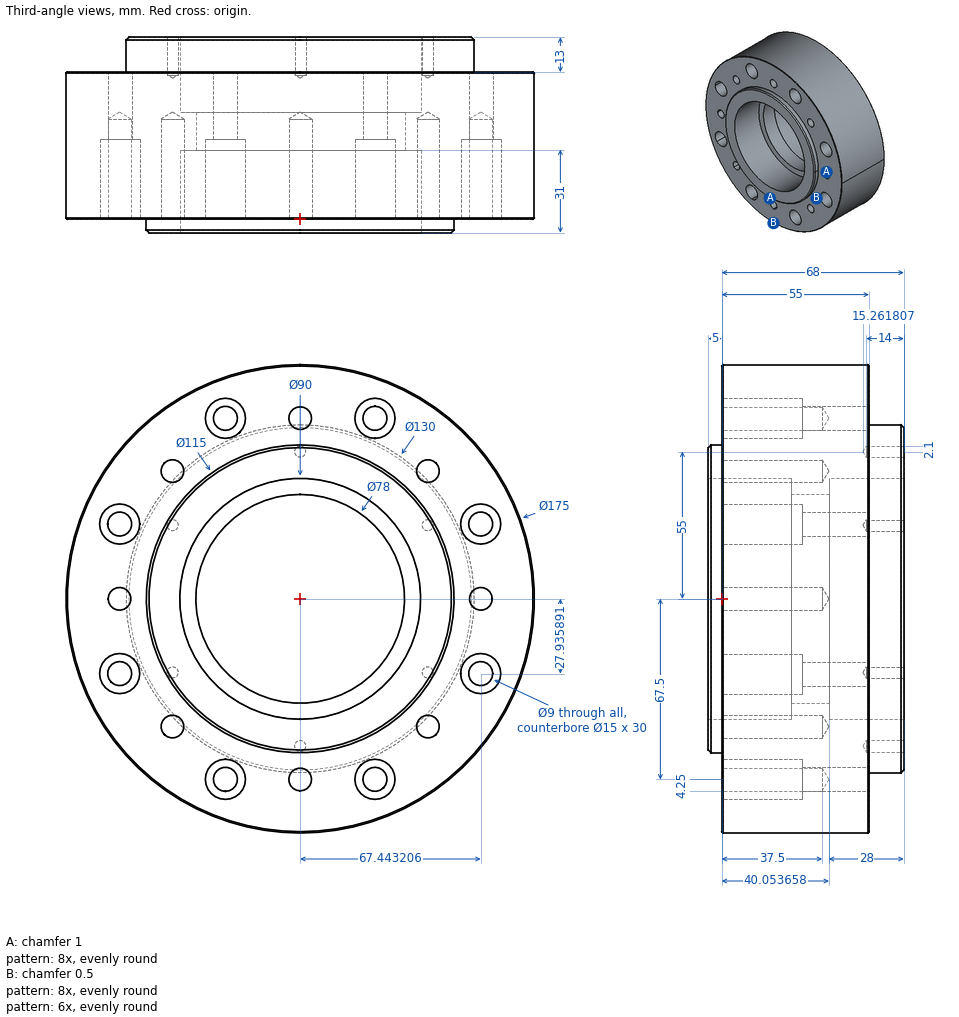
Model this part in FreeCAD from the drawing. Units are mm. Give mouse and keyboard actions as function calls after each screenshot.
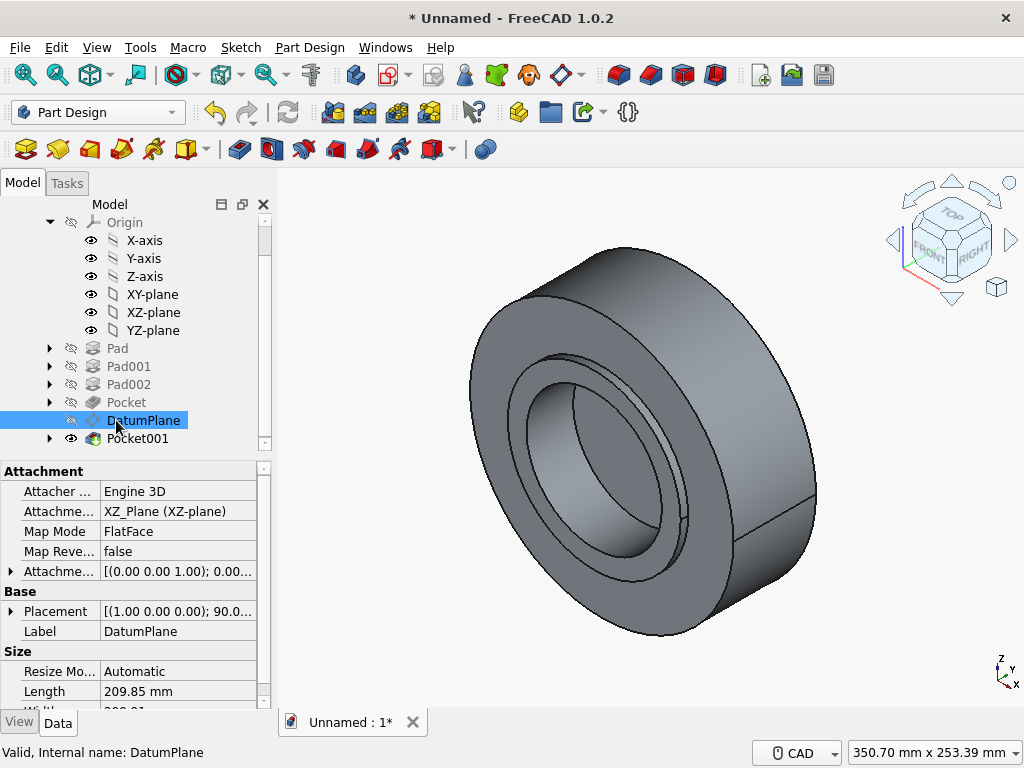
key(4)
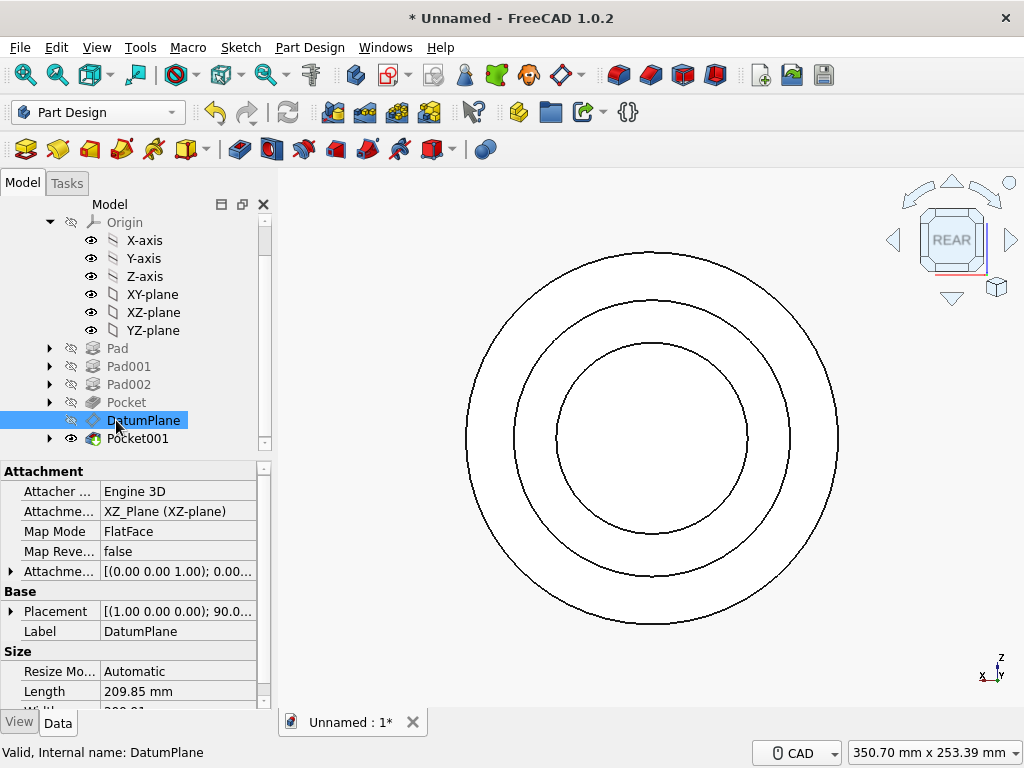
click(652, 437)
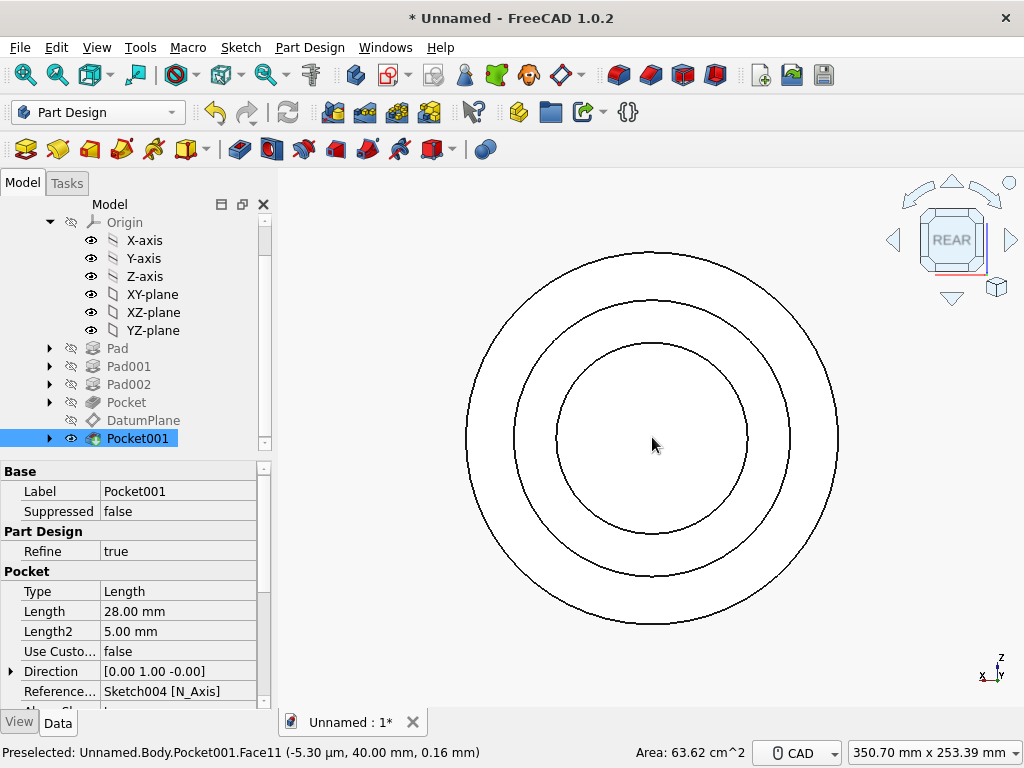
click(388, 76)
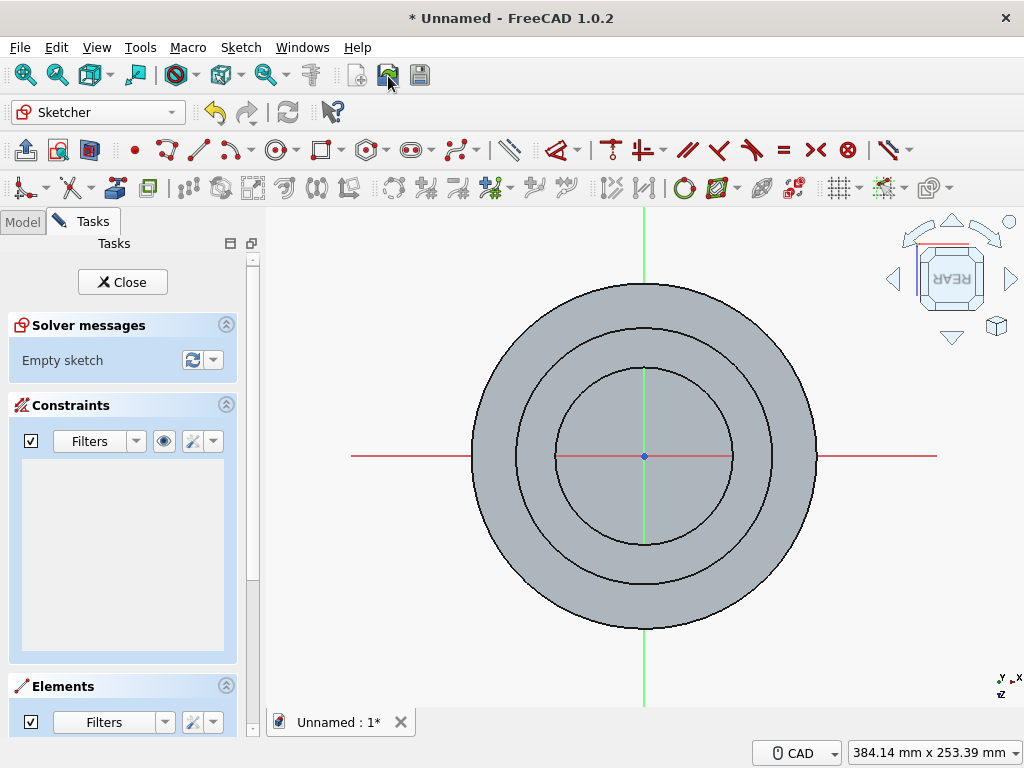
scroll(699, 456, up, 4)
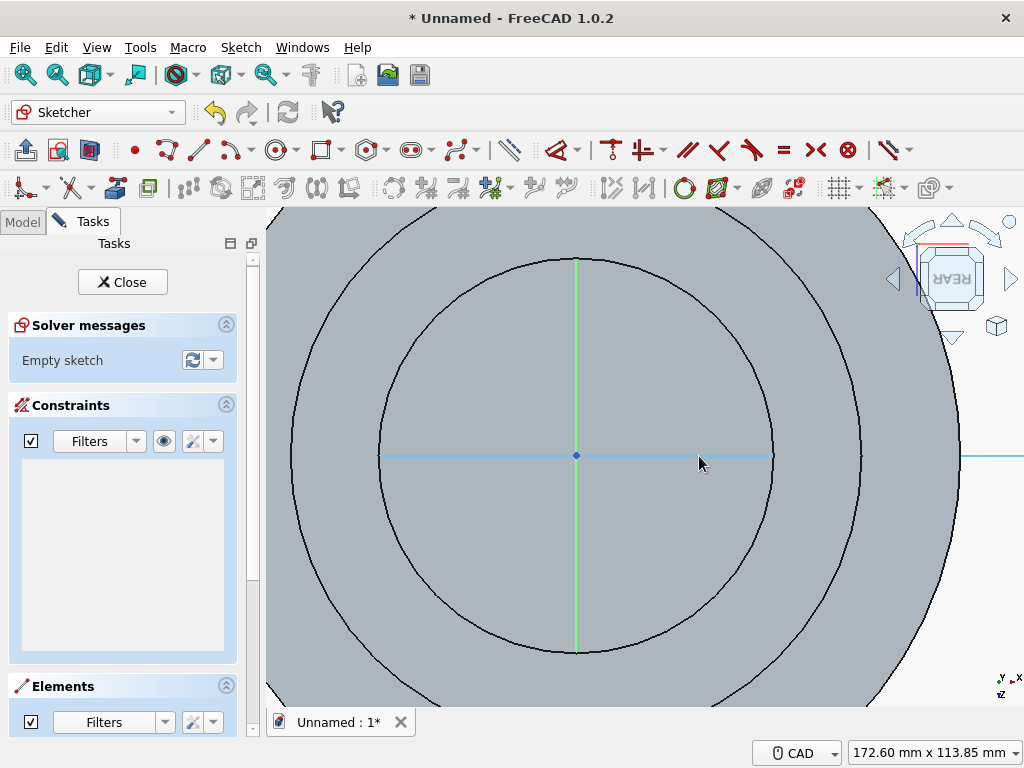
click(276, 150)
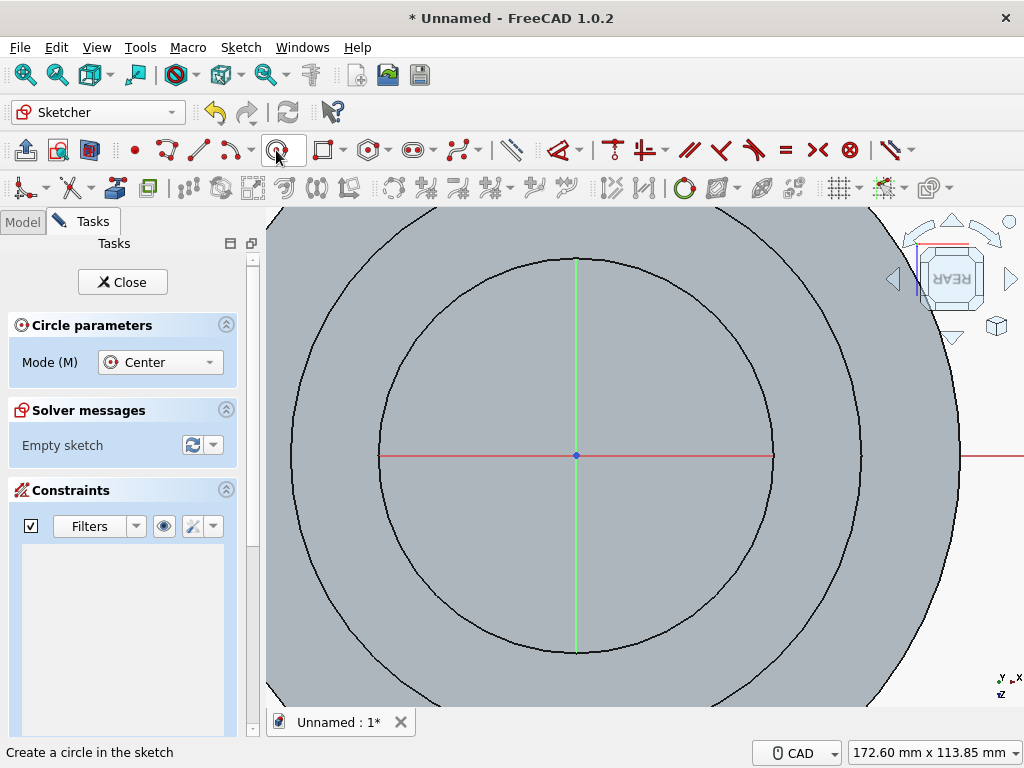
click(576, 456)
click(697, 335)
key(Escape)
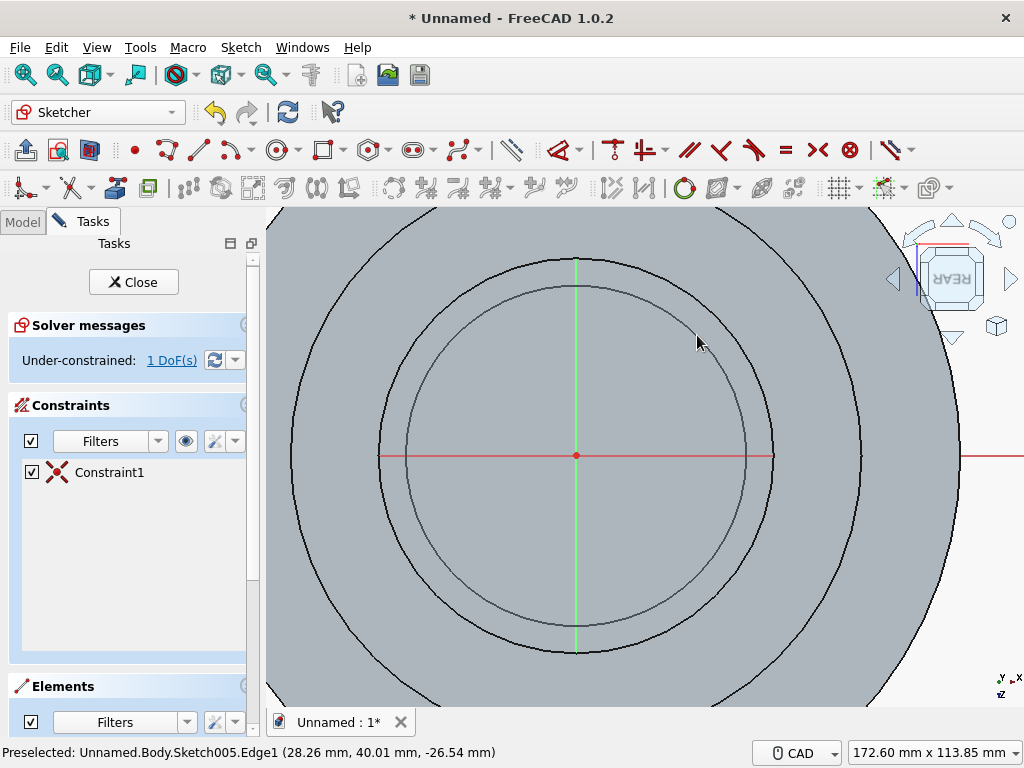
click(558, 150)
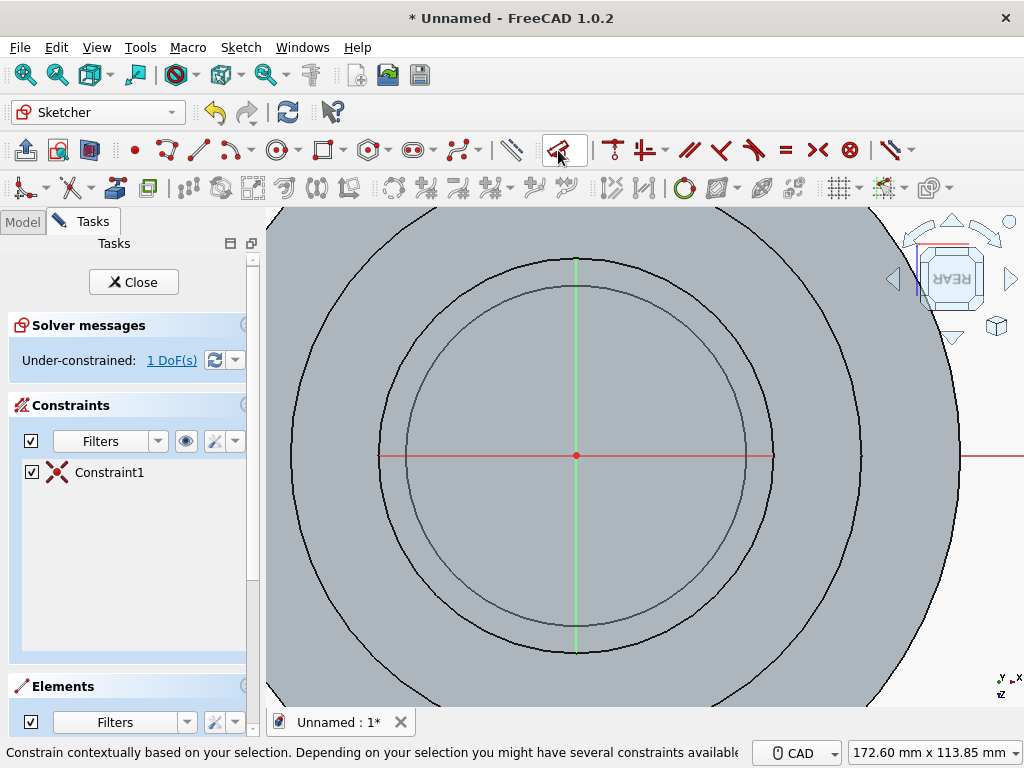
click(696, 335)
click(719, 312)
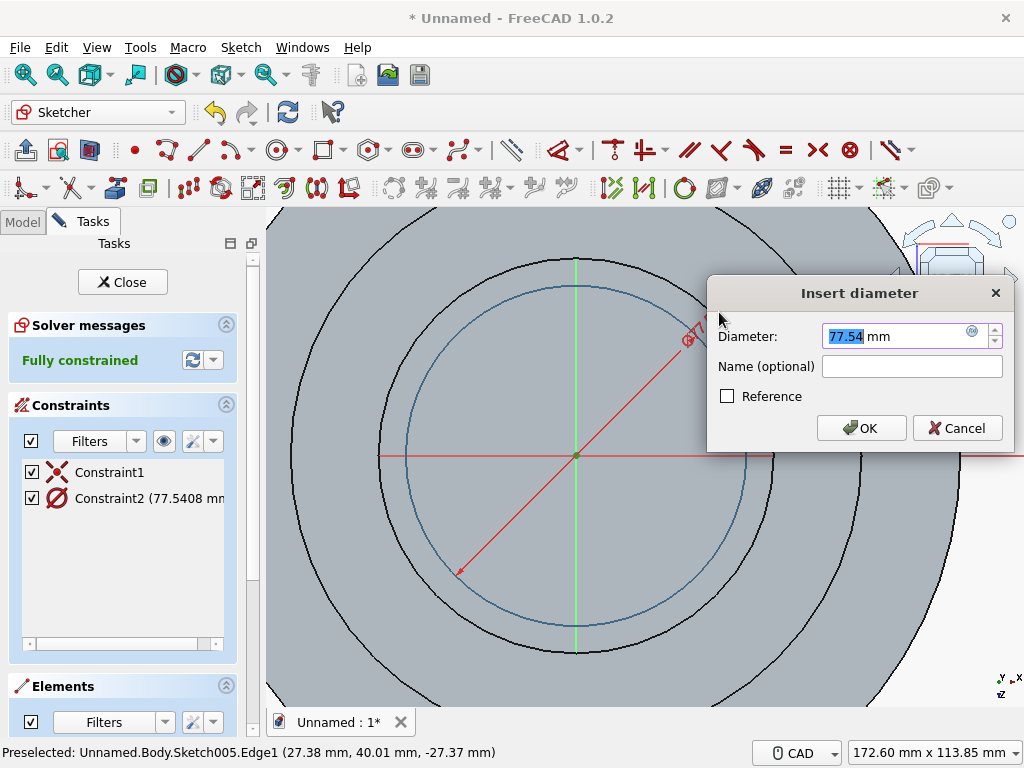
text(78)
key(Return)
key(Escape)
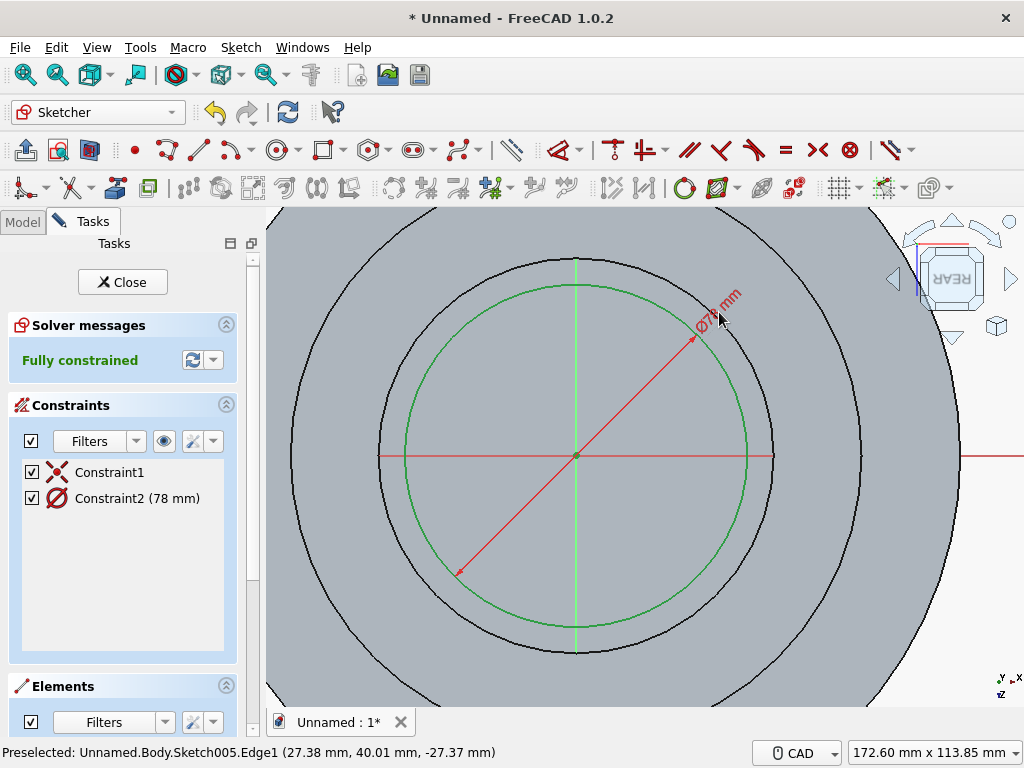
click(123, 282)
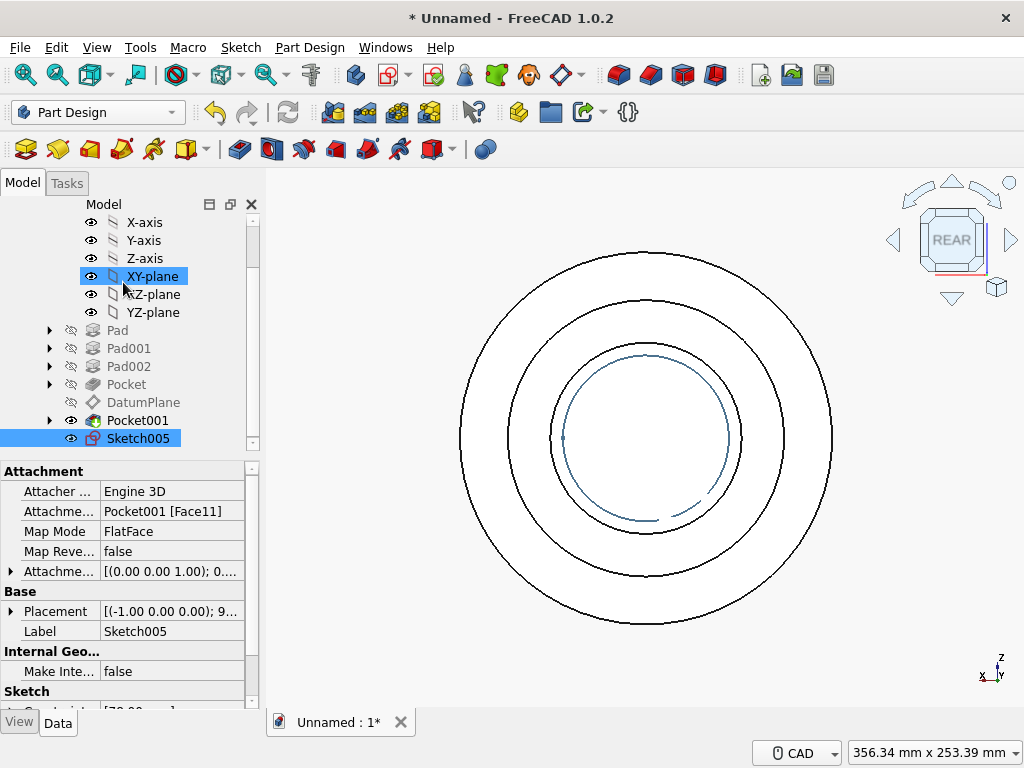
click(240, 150)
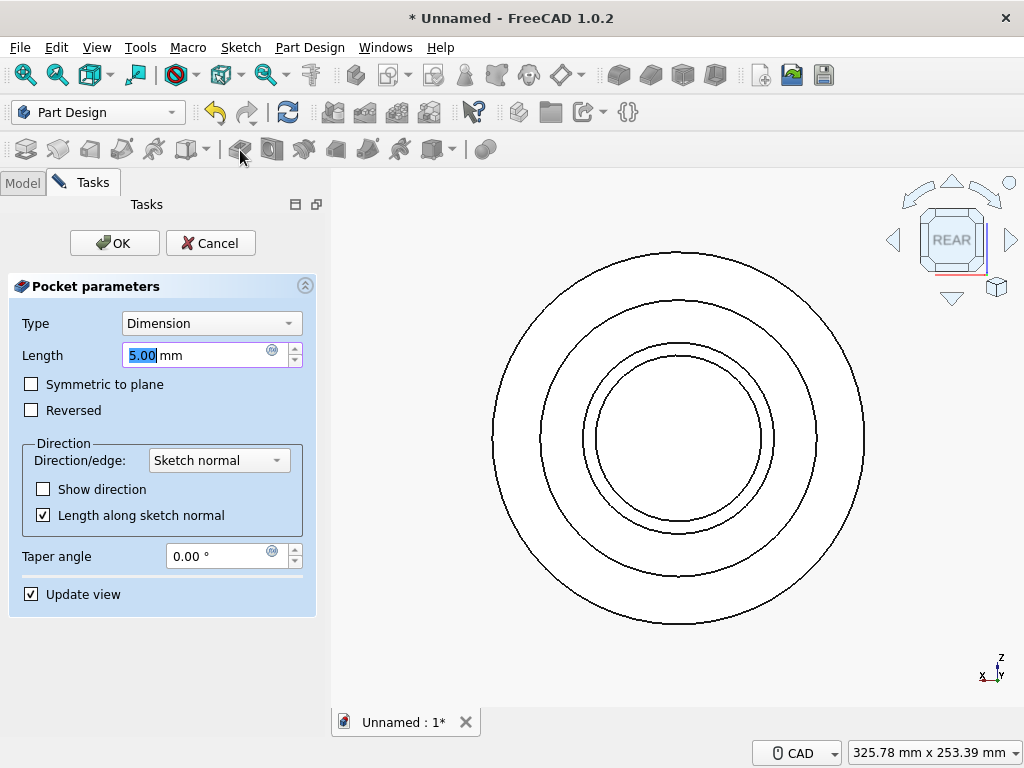
click(212, 324)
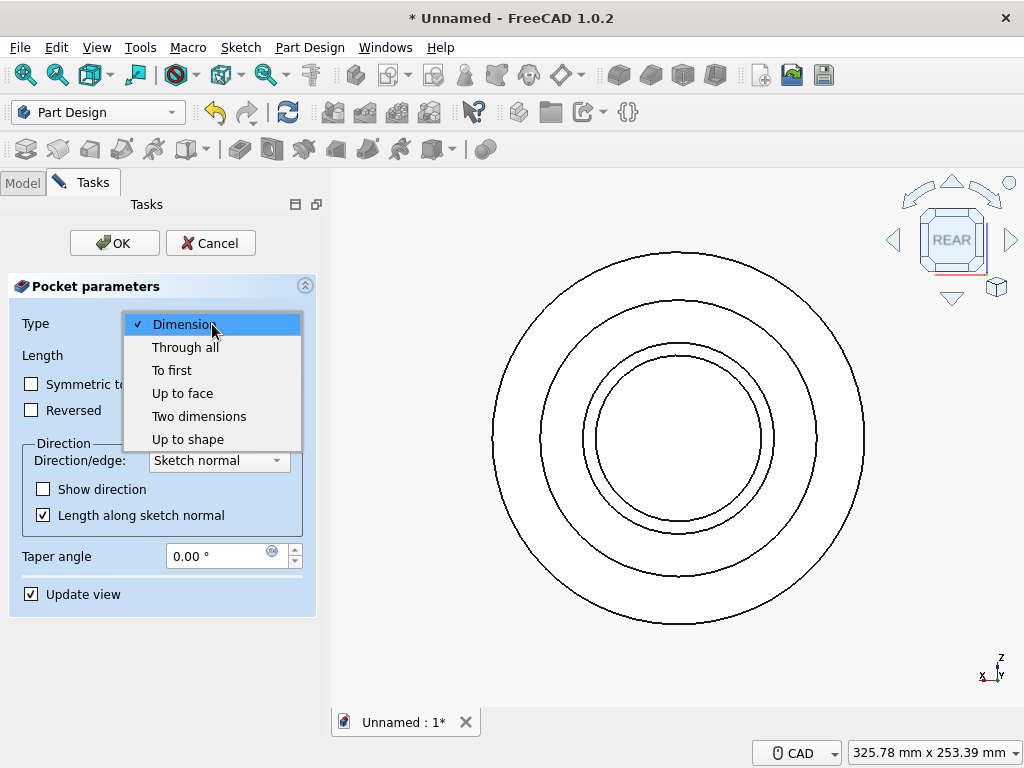
click(212, 348)